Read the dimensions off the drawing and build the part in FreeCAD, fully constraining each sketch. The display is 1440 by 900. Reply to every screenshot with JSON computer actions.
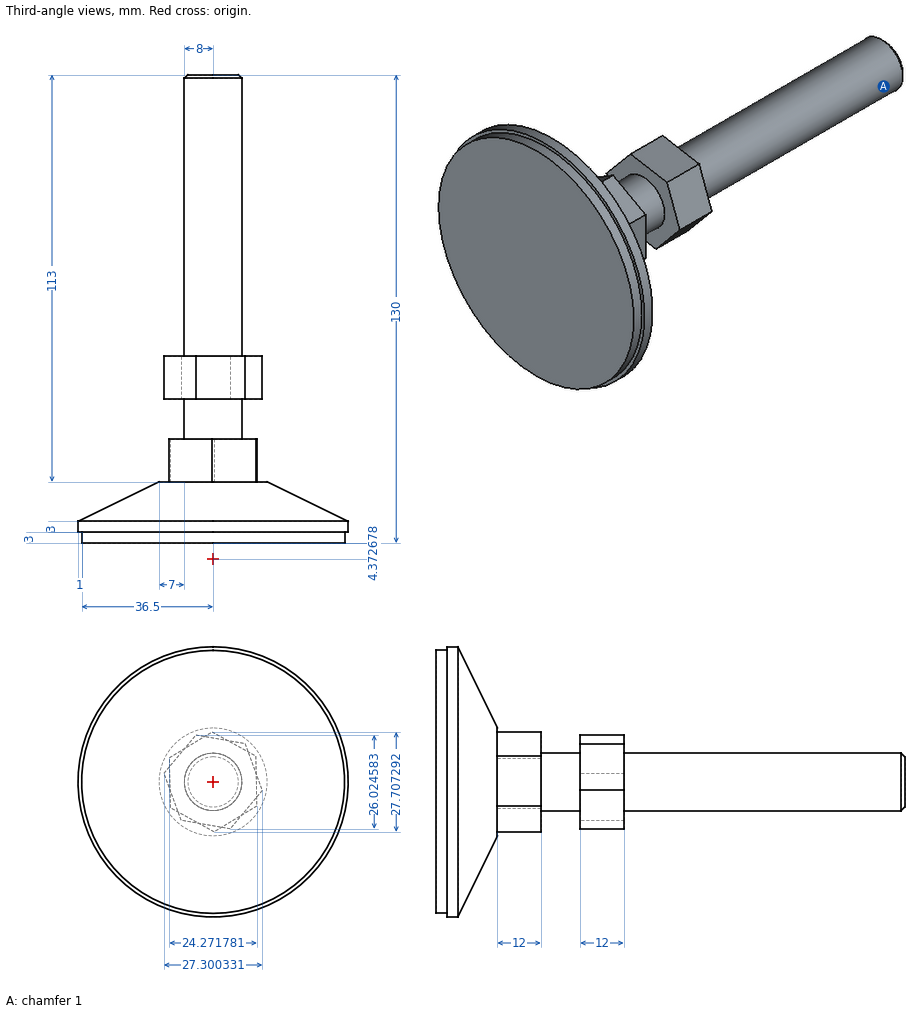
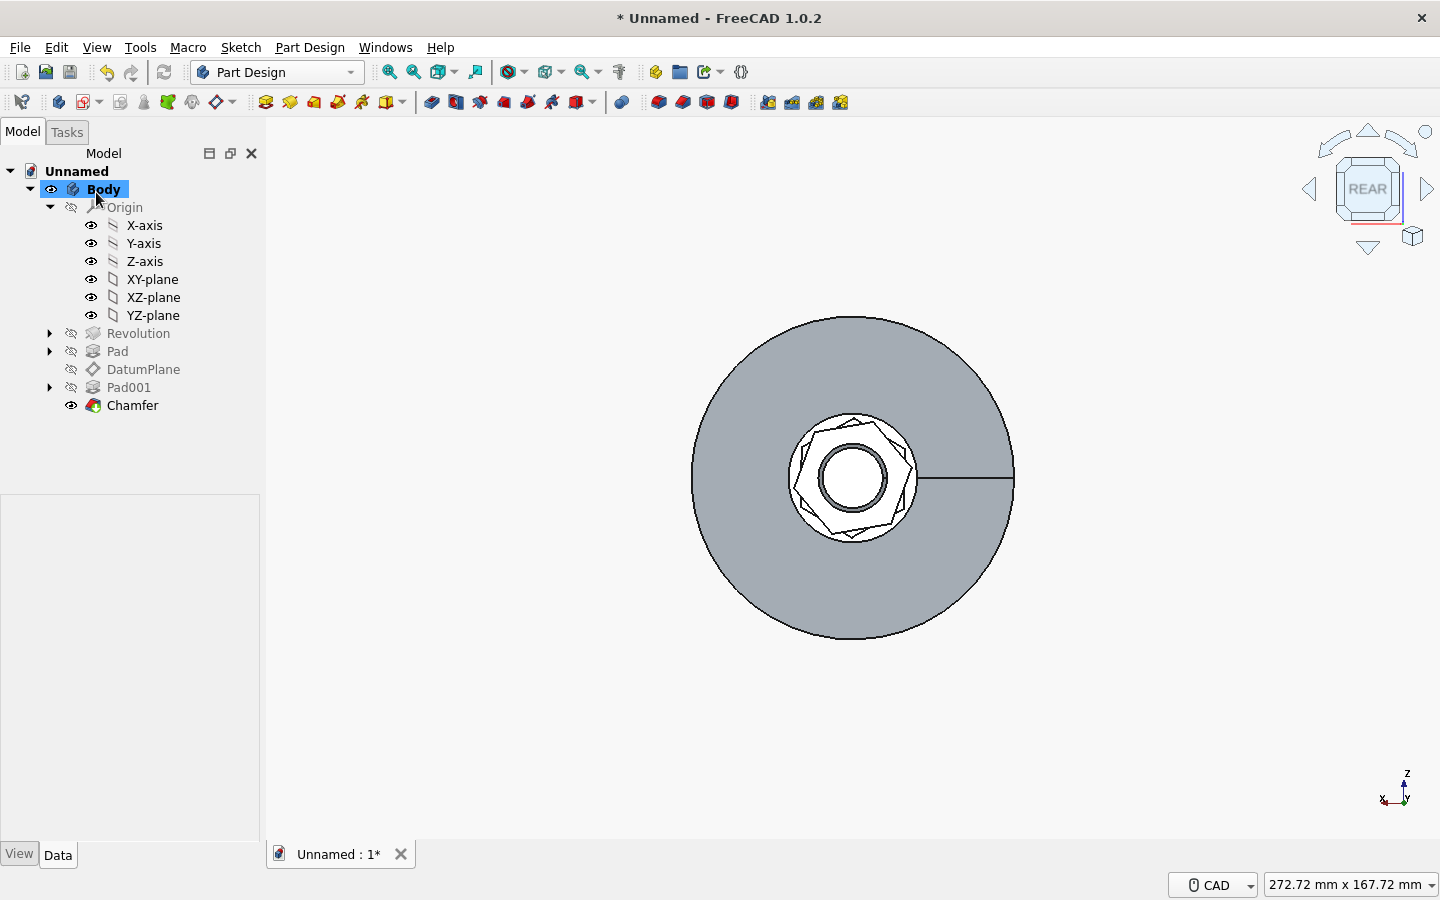
{"action": "key", "text": "0"}